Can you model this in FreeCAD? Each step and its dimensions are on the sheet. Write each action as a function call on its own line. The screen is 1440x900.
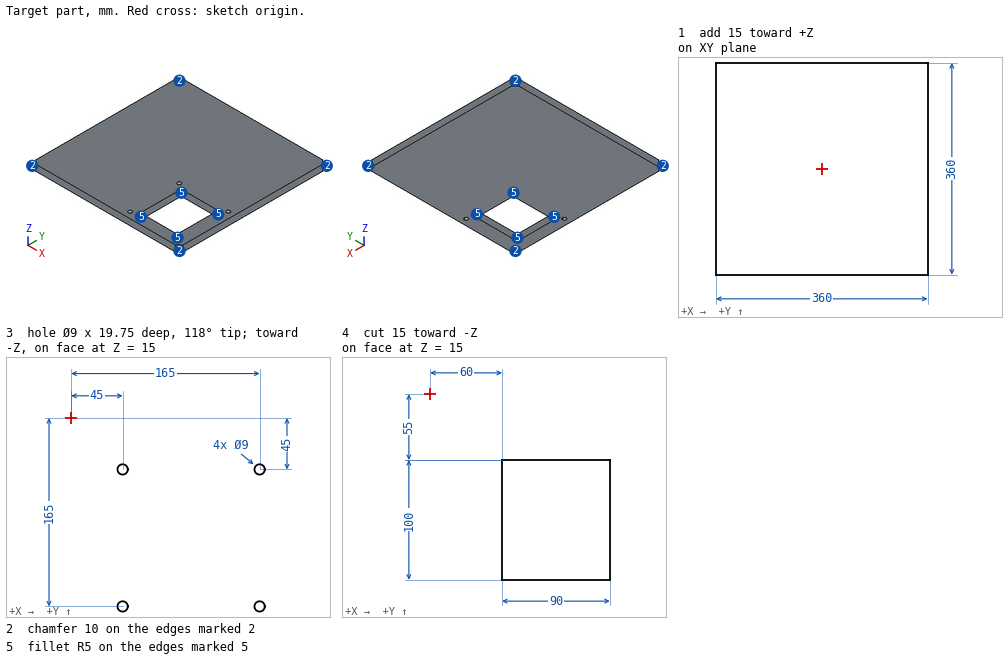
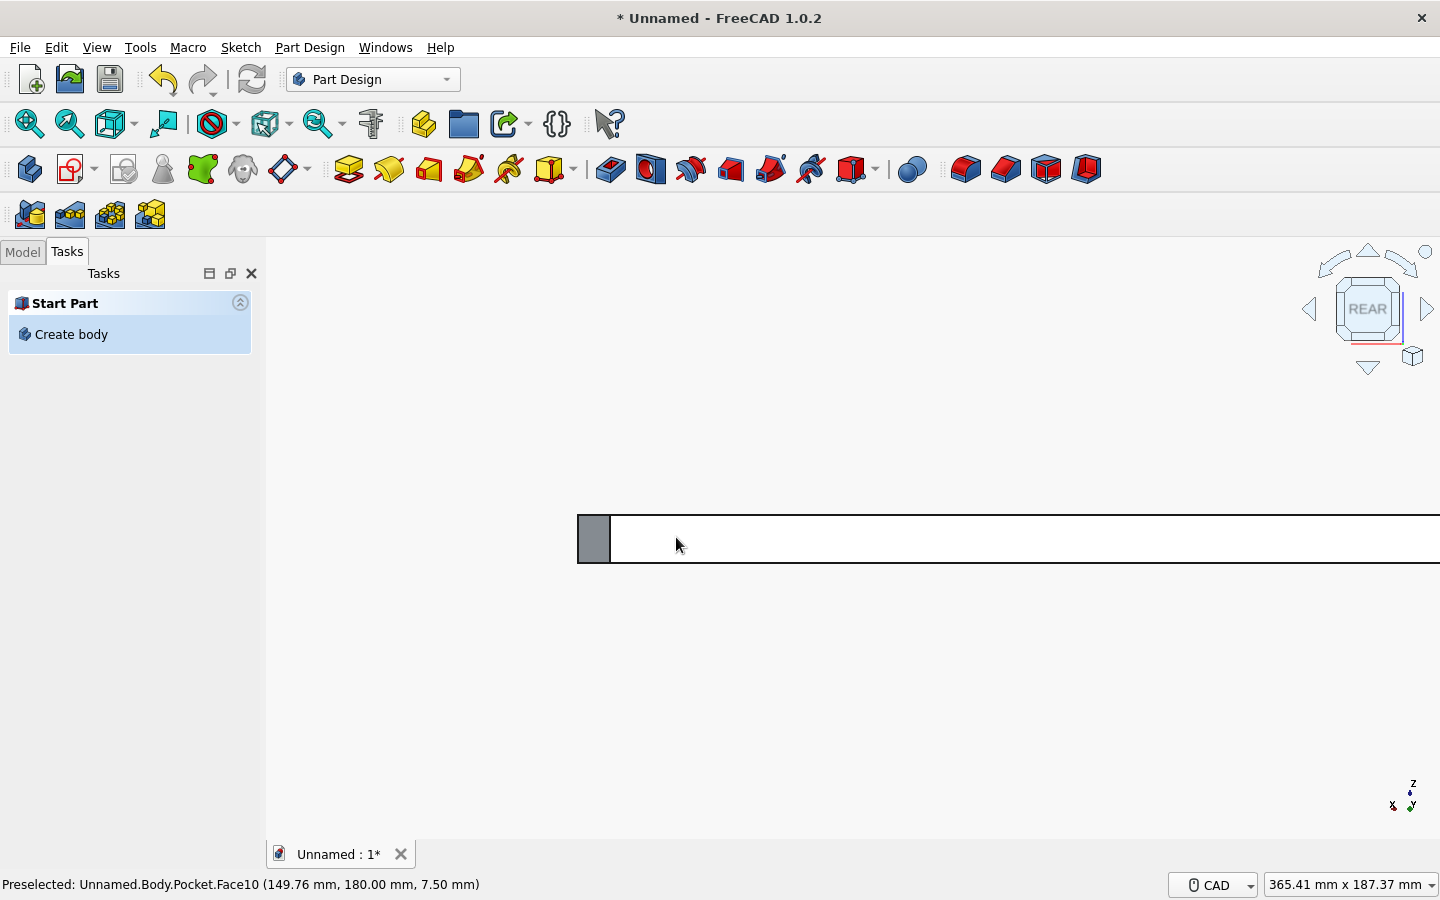
key(v)
key(f)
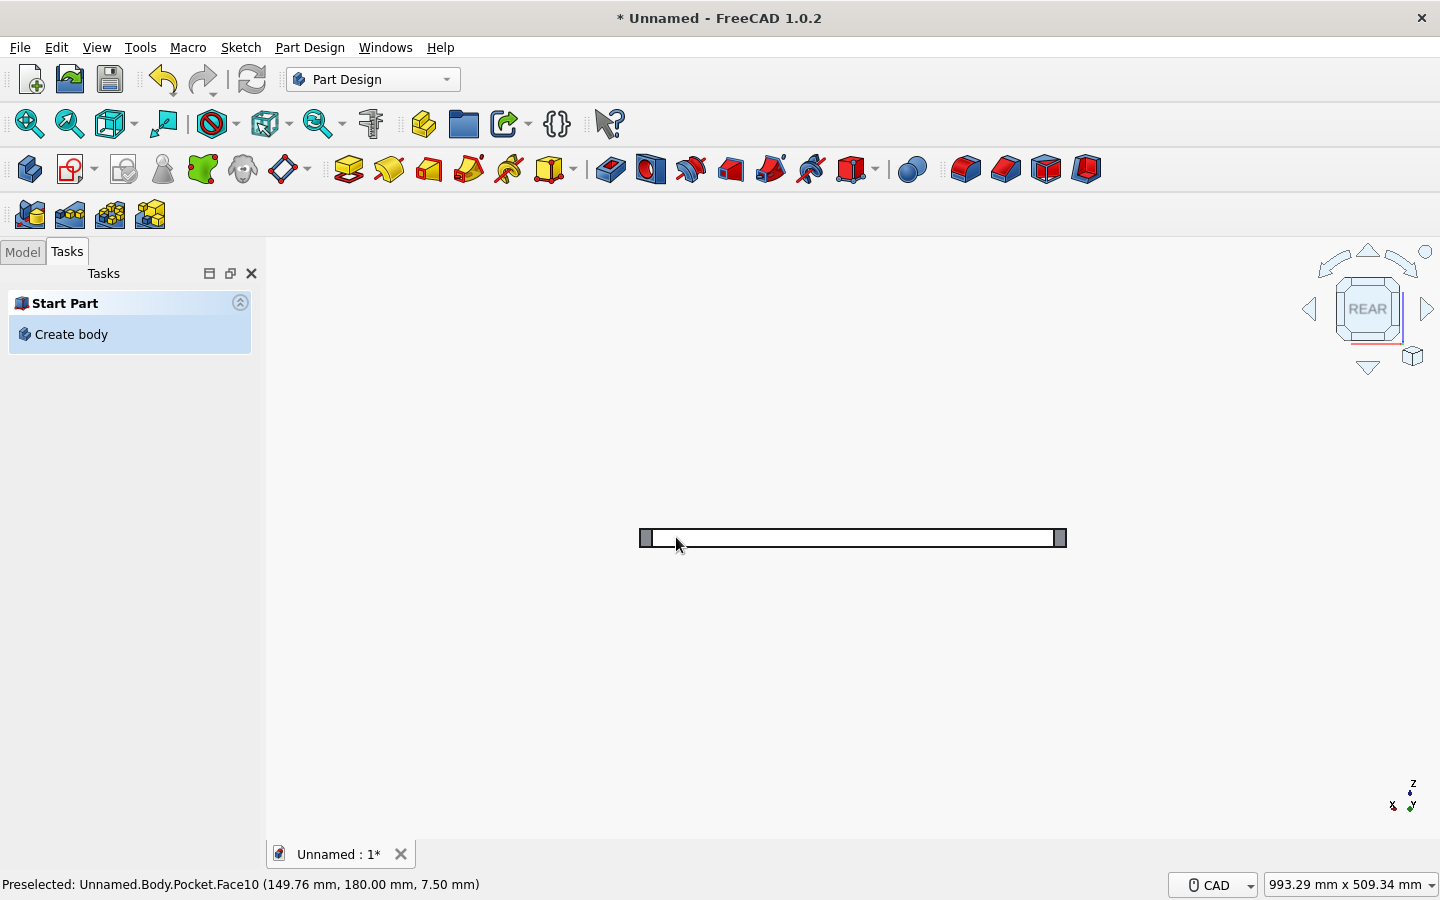
key(6)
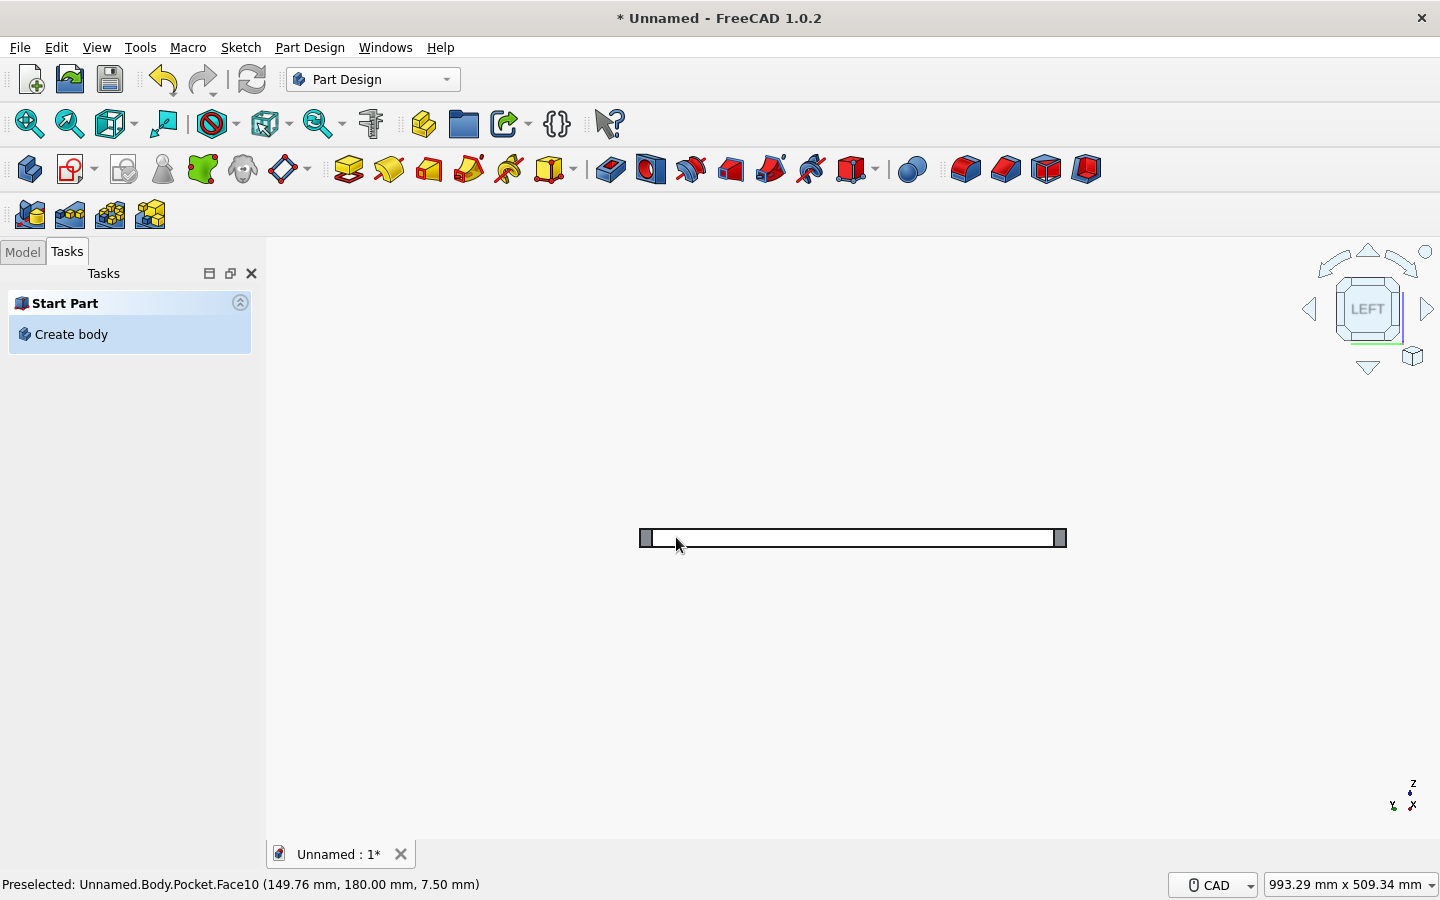
key(v)
key(f)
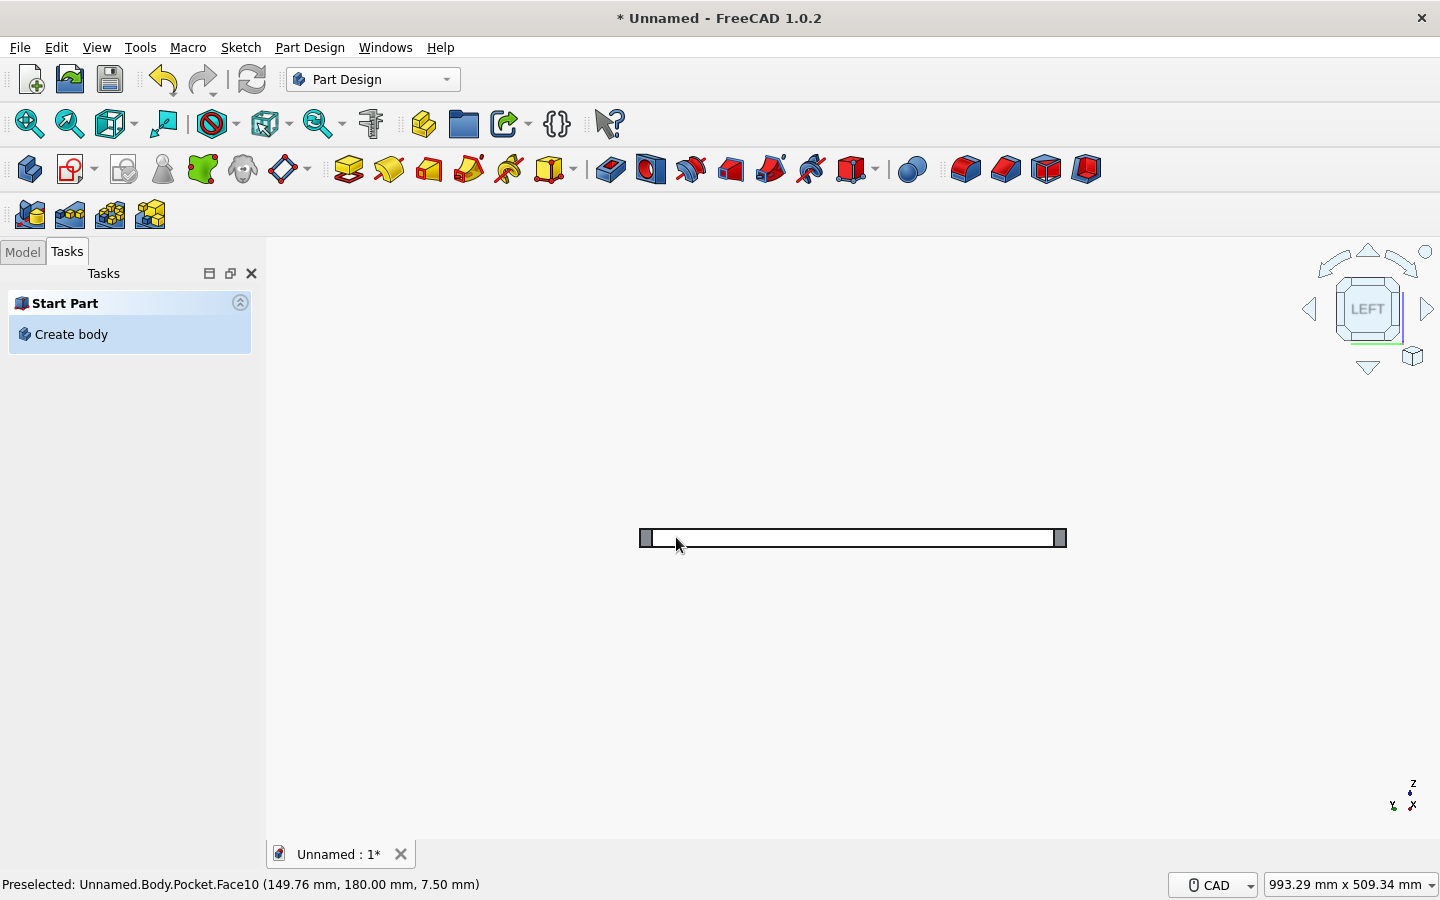
scroll(918, 537, up, 5)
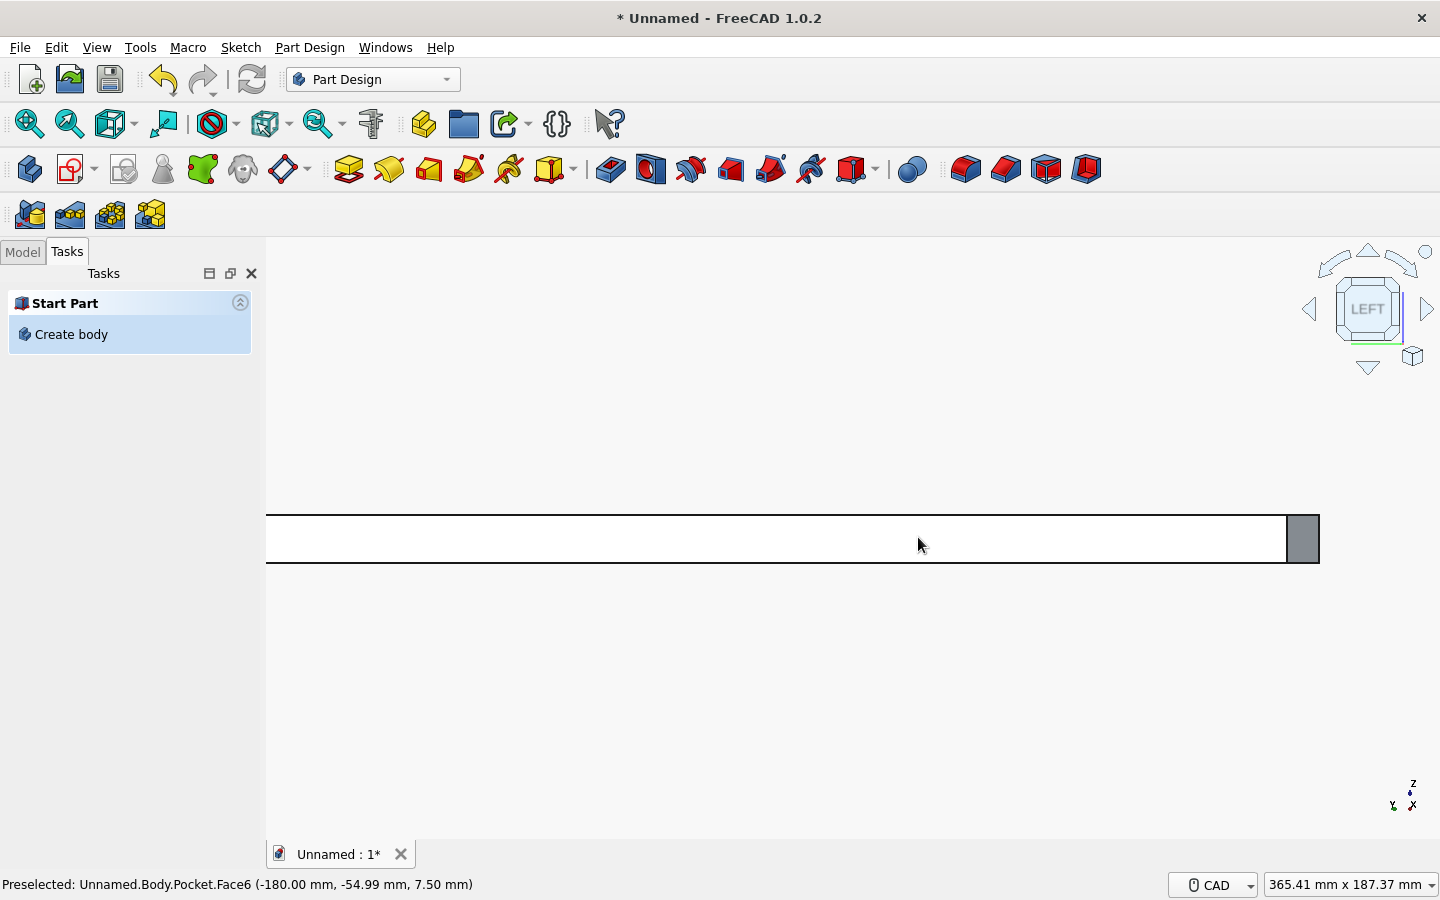
click(30, 124)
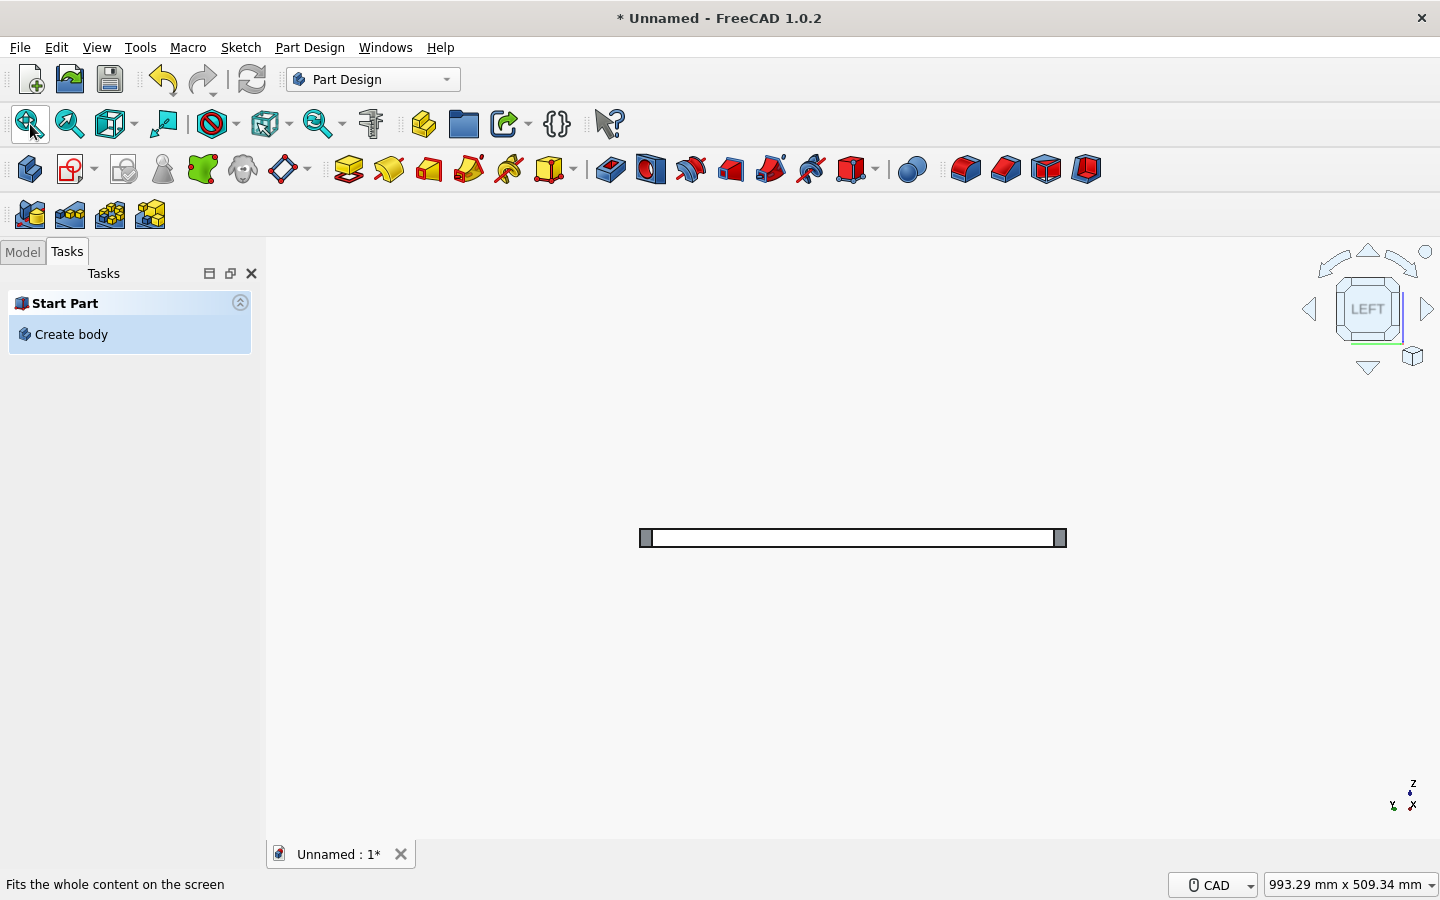
key(v)
key(3)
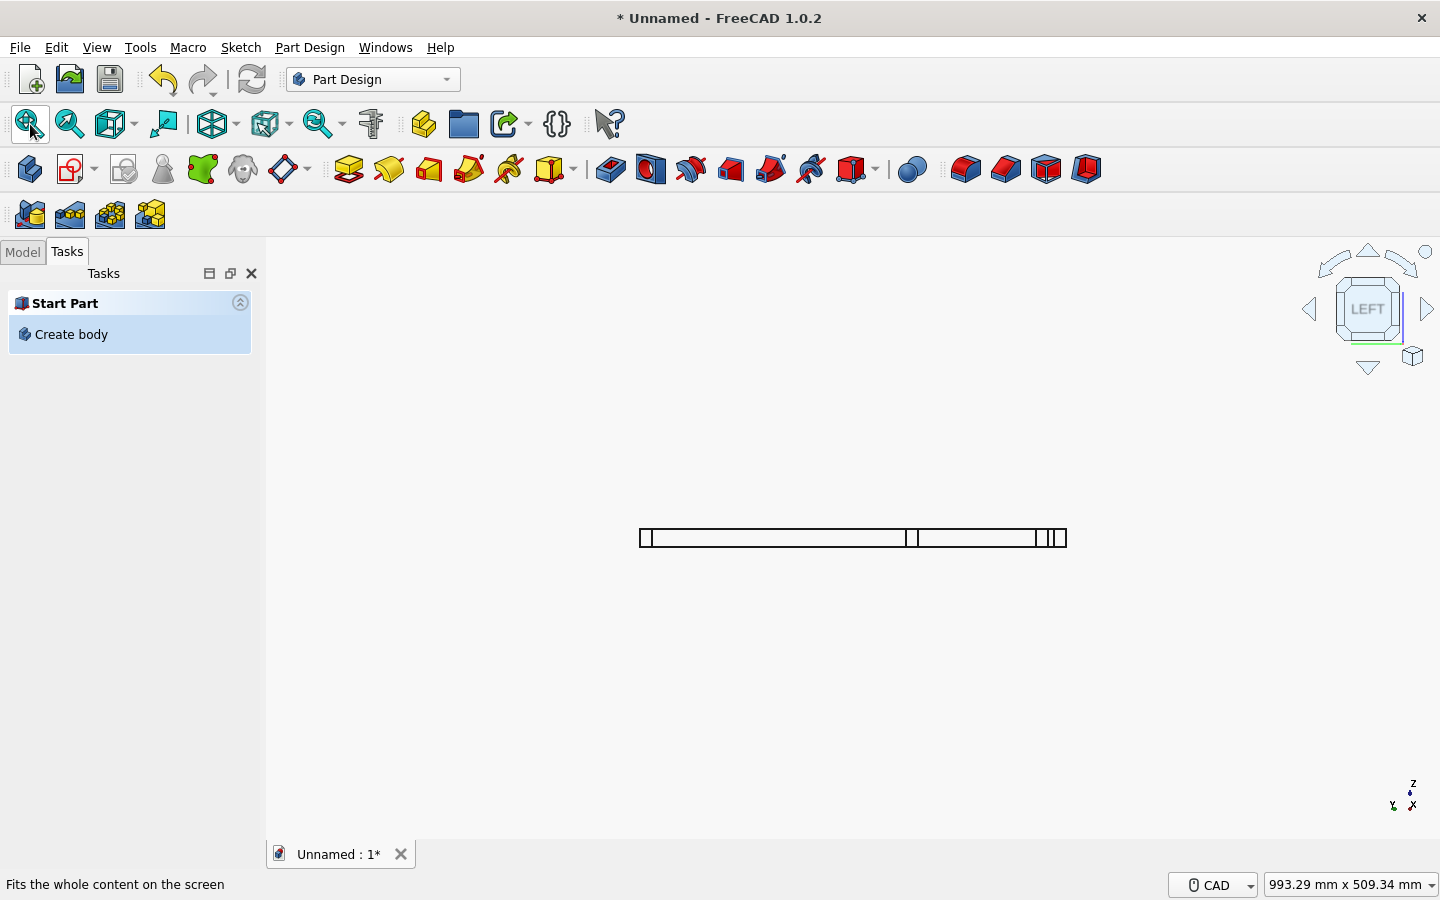
key(0)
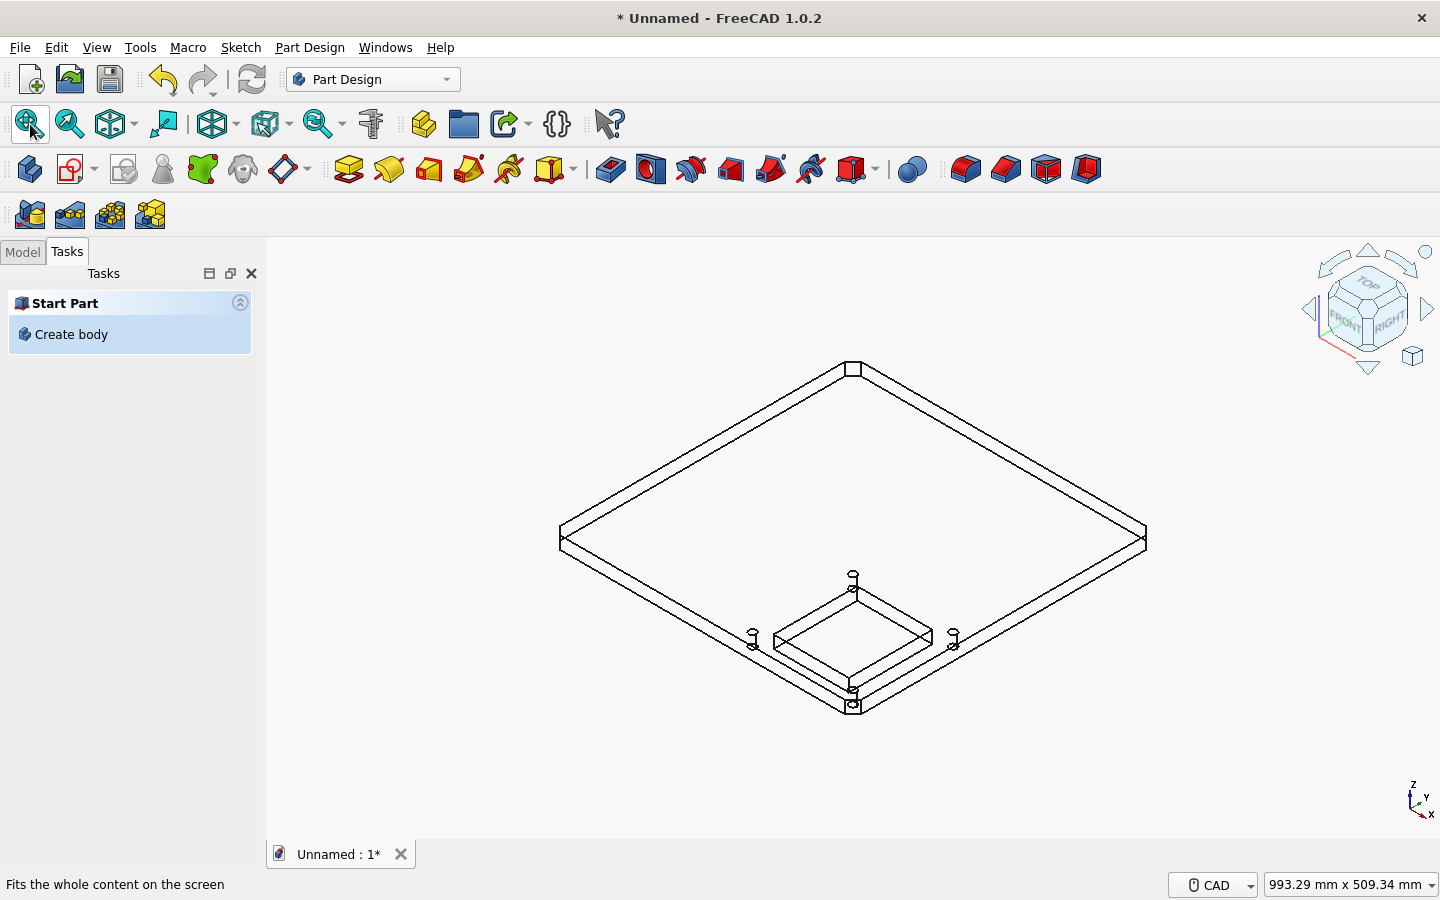
click(932, 637)